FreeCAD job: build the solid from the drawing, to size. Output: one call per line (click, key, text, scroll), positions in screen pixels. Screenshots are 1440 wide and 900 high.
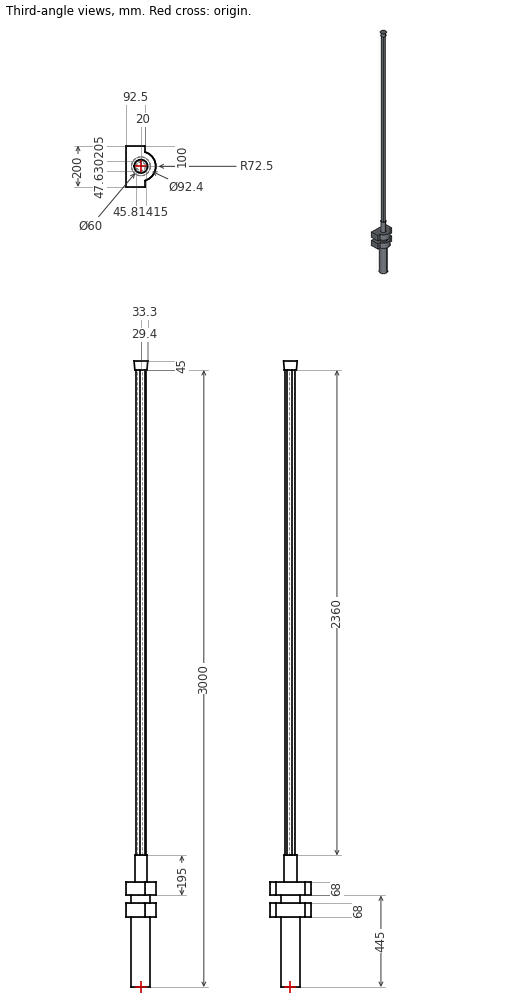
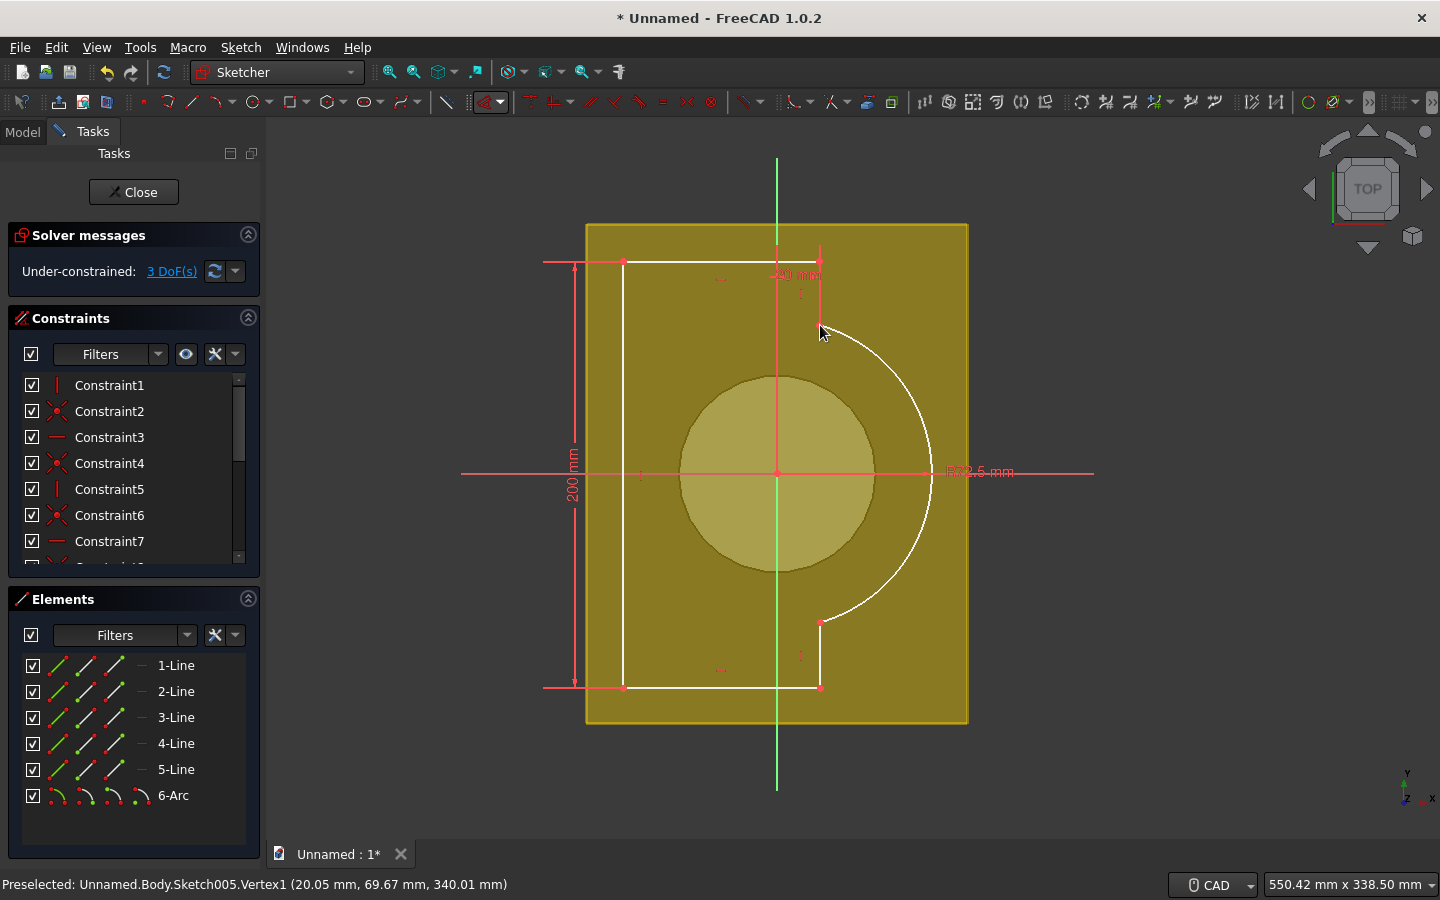
click(820, 688)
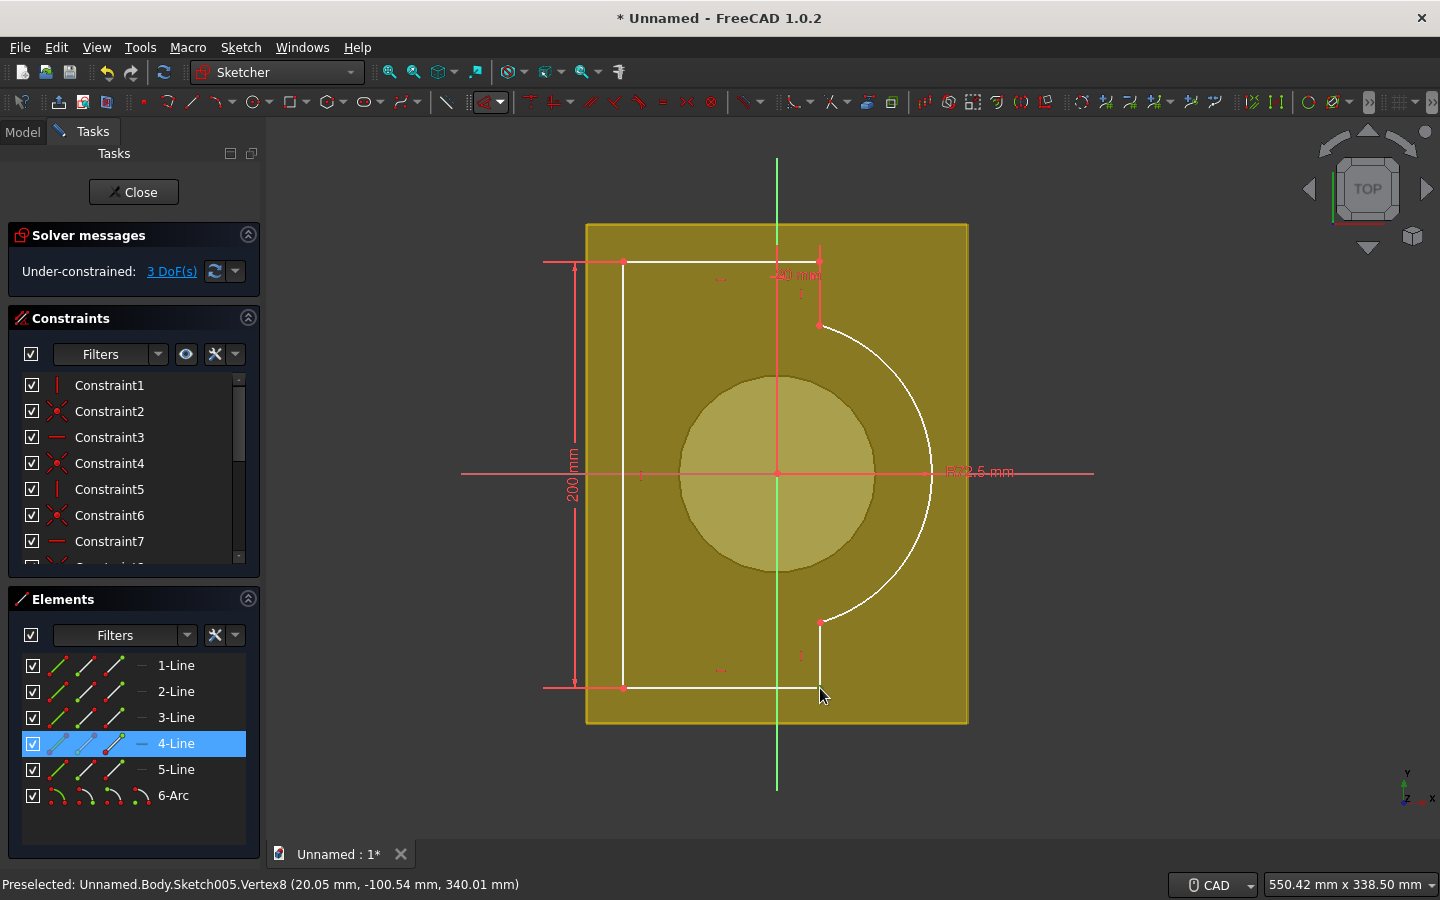
key(l)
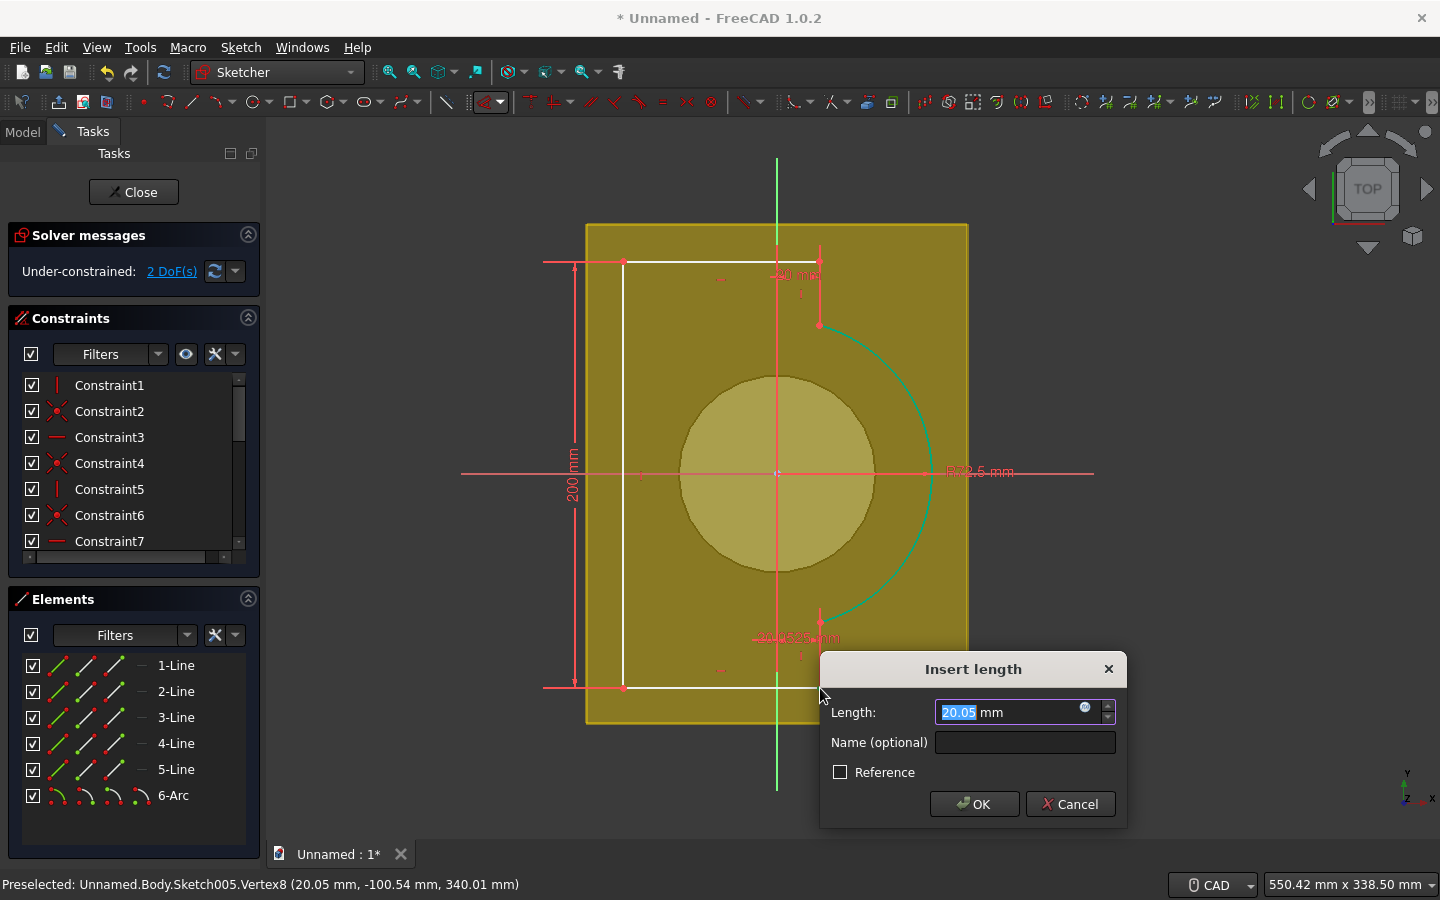
text(20)
key(Return)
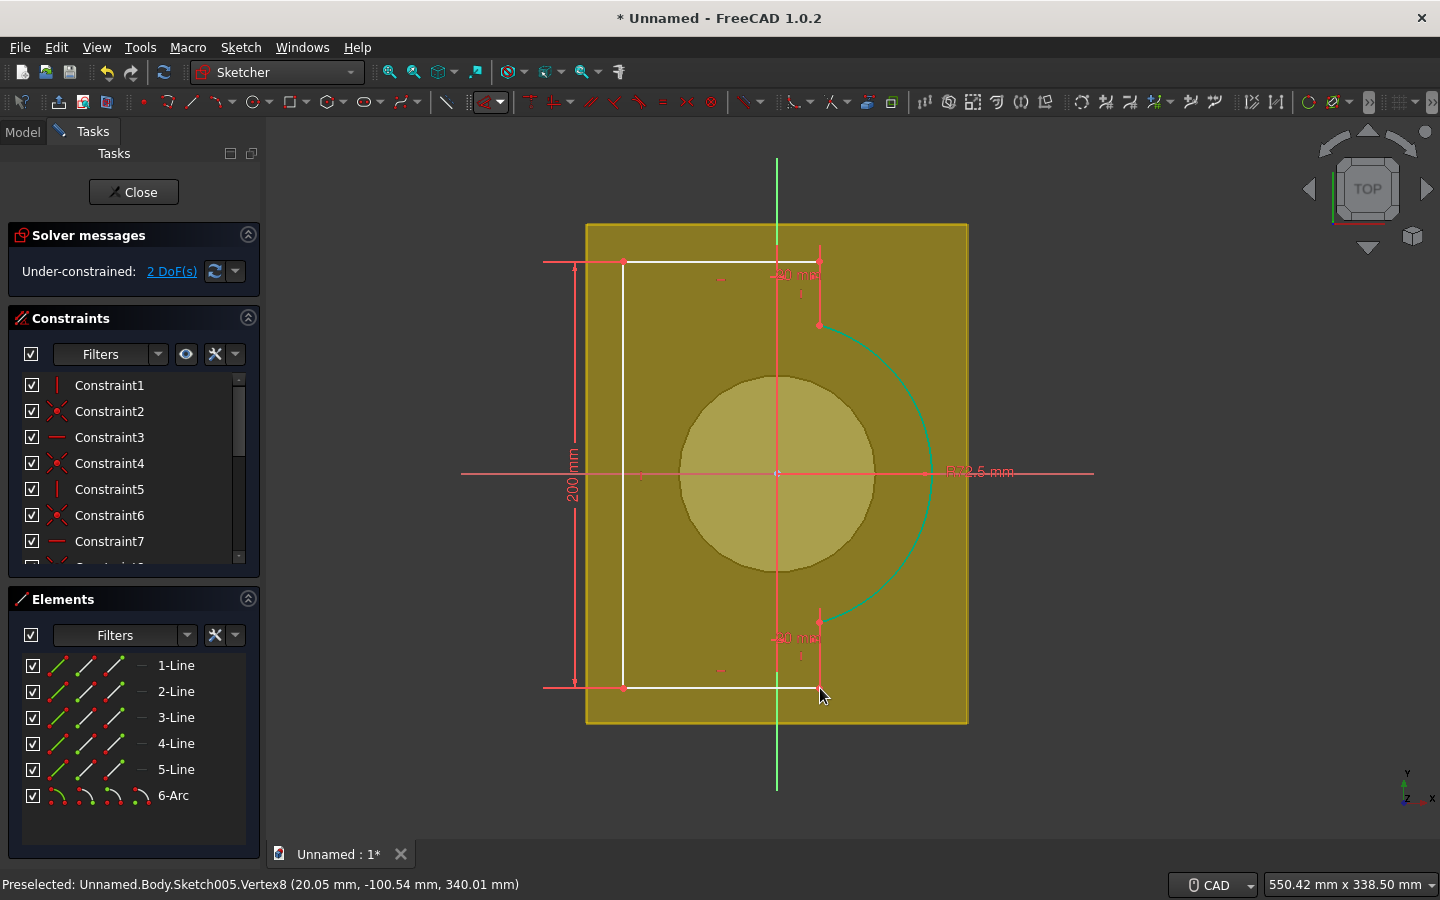
click(761, 262)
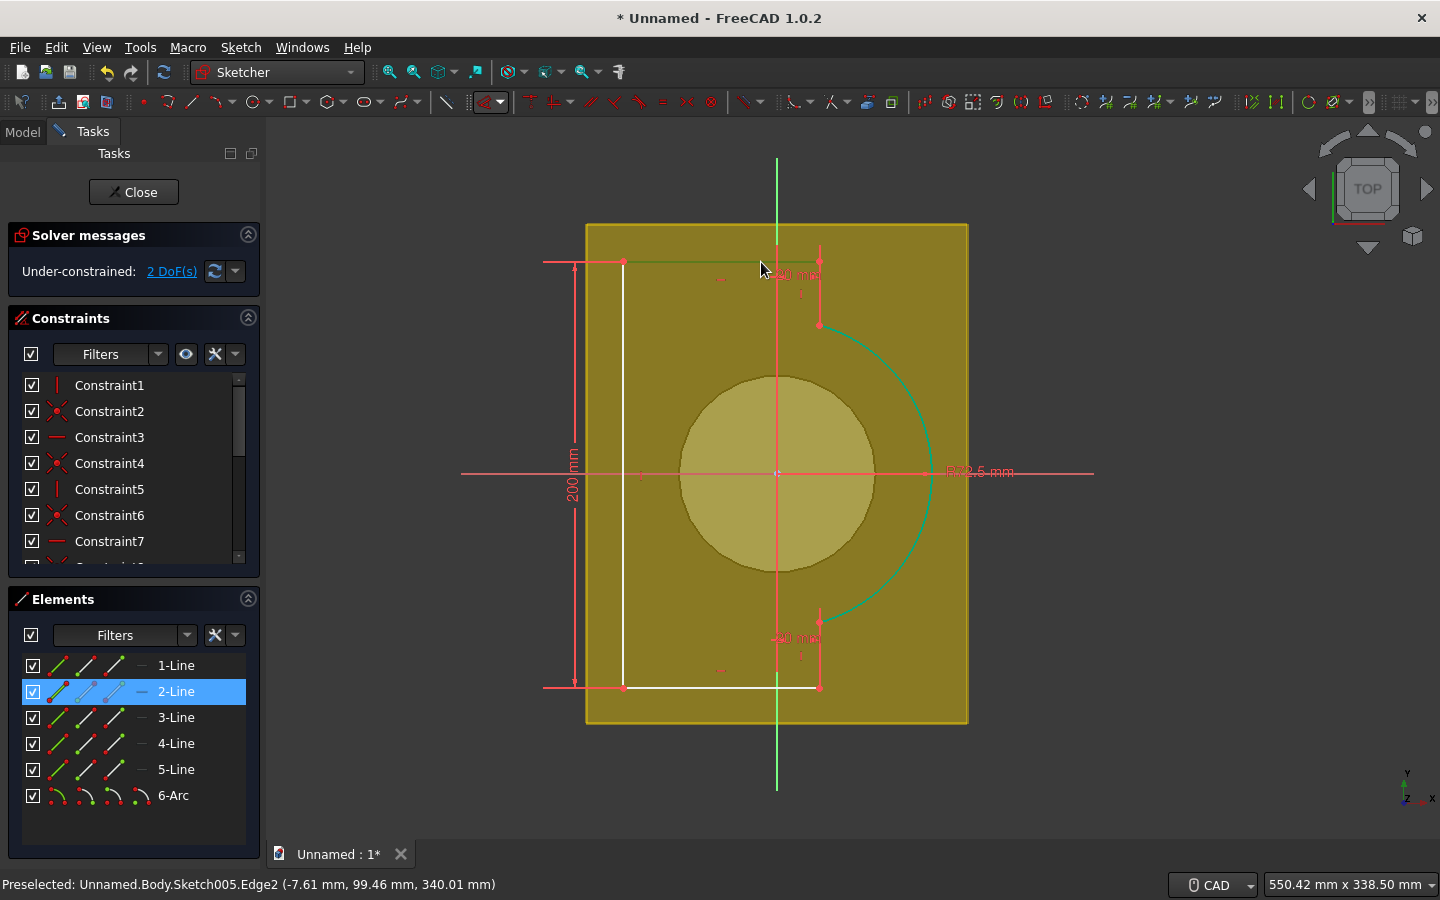
key(l)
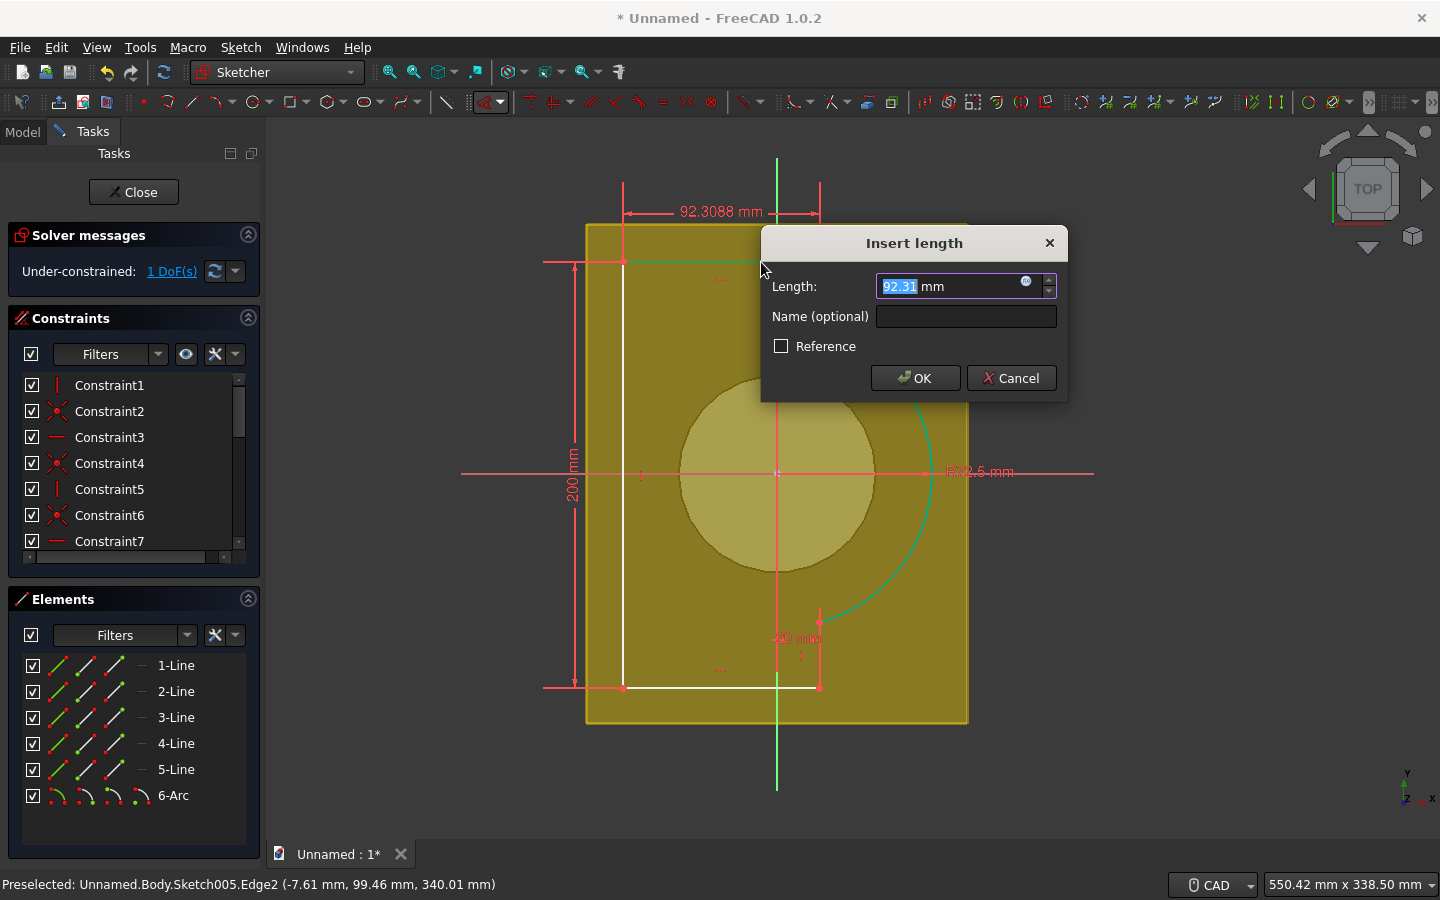
text(92.5)
key(Return)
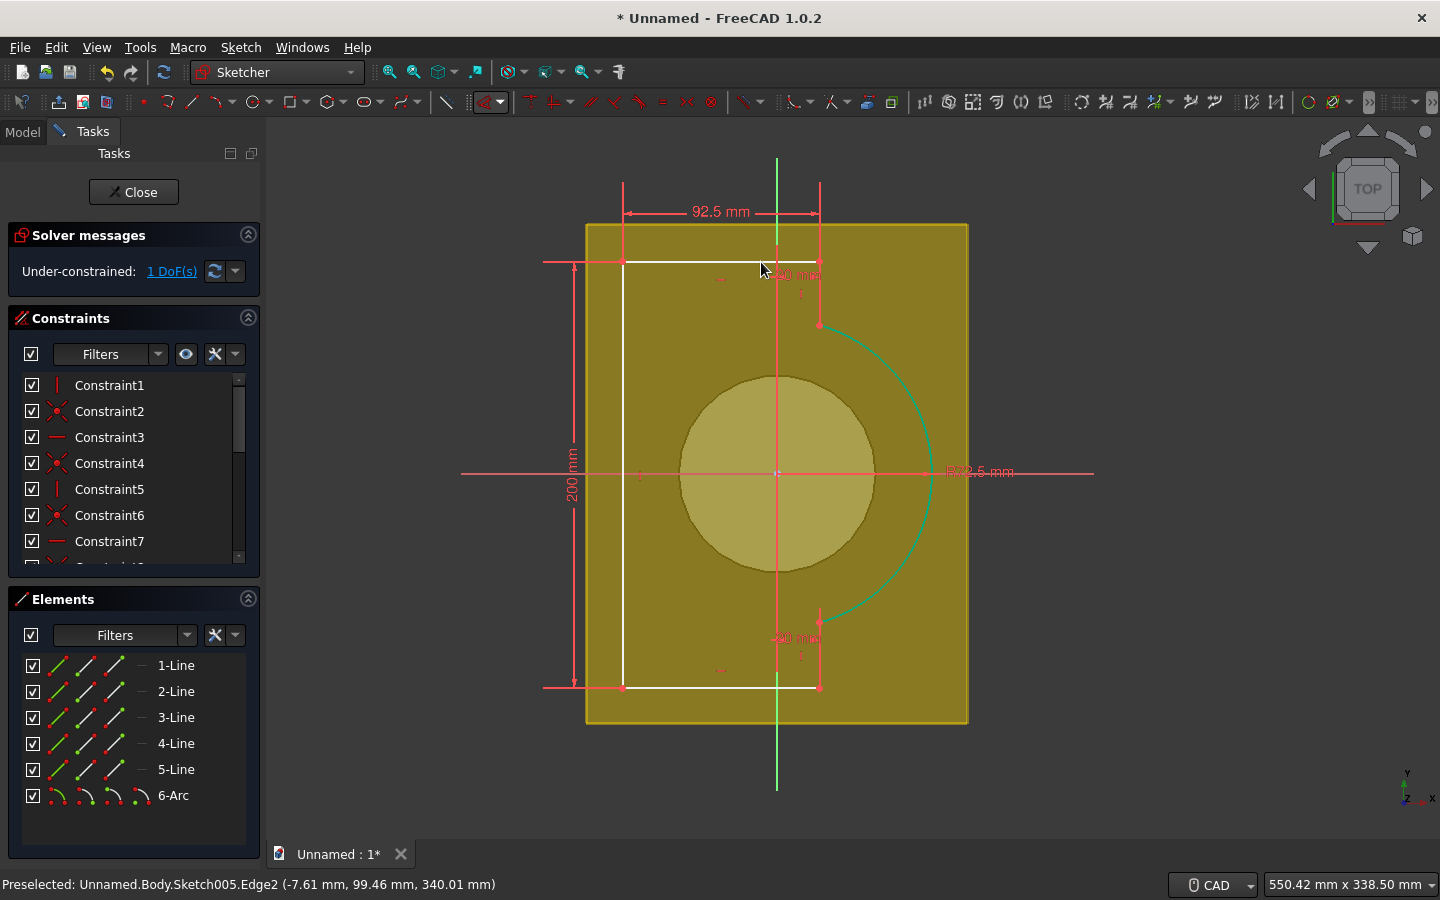
click(820, 262)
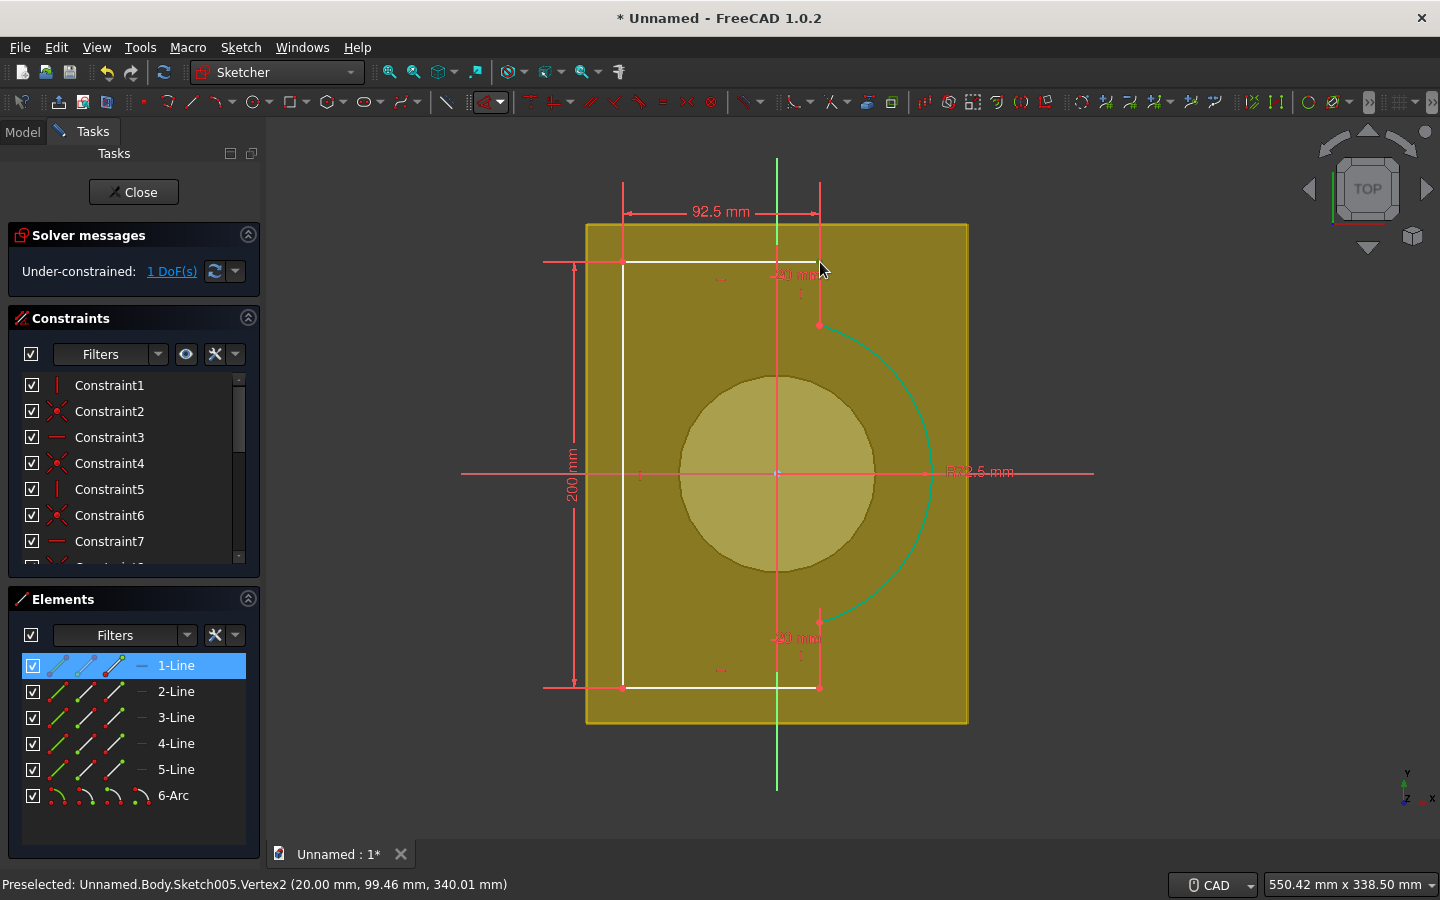
key(i)